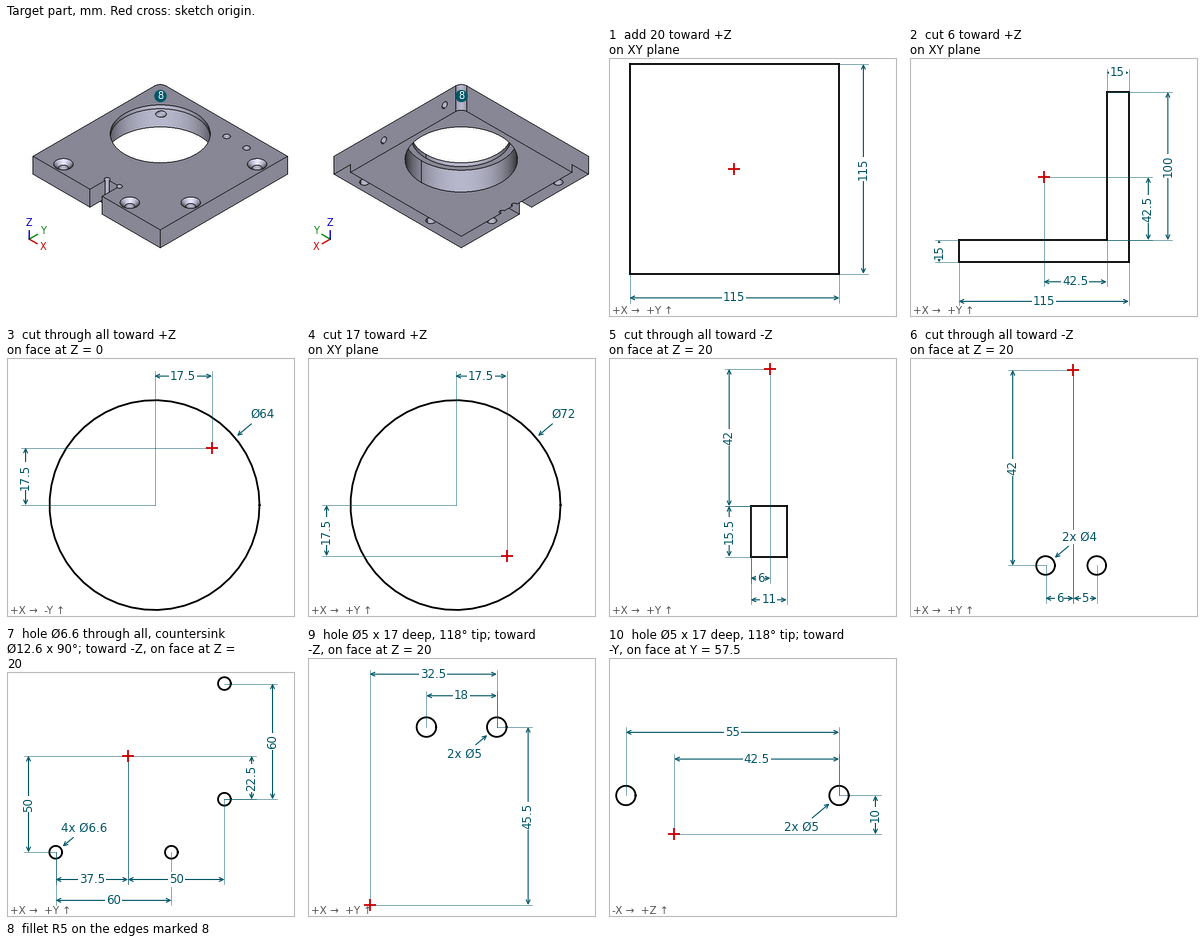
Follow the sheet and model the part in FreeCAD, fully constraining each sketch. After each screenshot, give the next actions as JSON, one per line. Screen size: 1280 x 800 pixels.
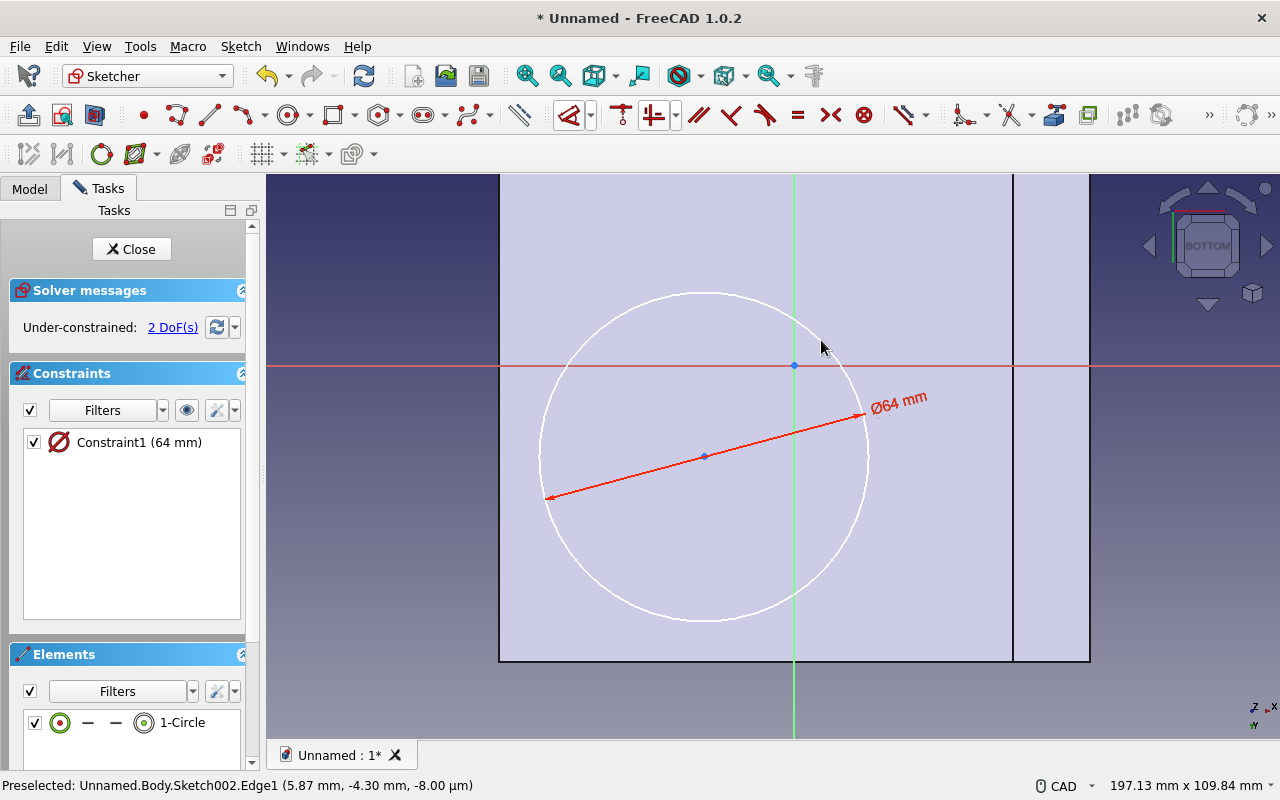
{"action": "left_click", "coordinate": [704, 457]}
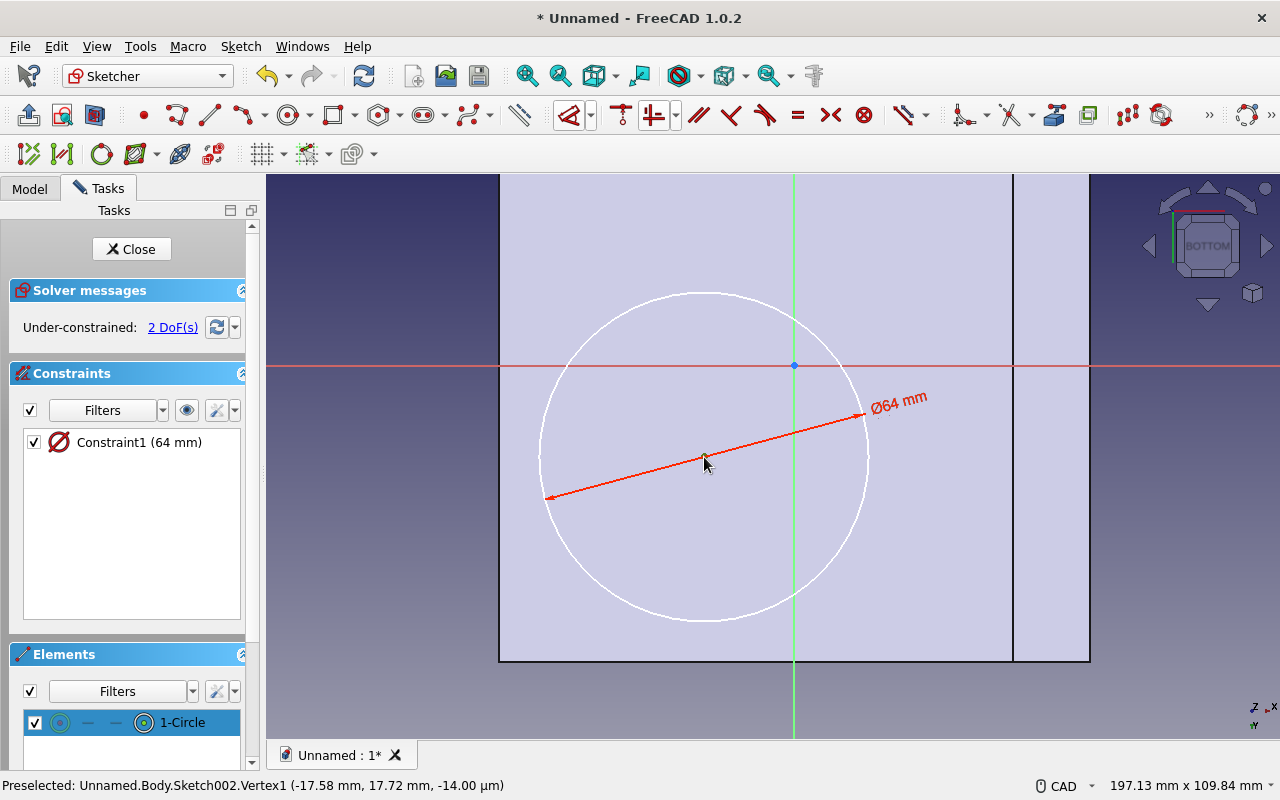
{"action": "key", "text": "l"}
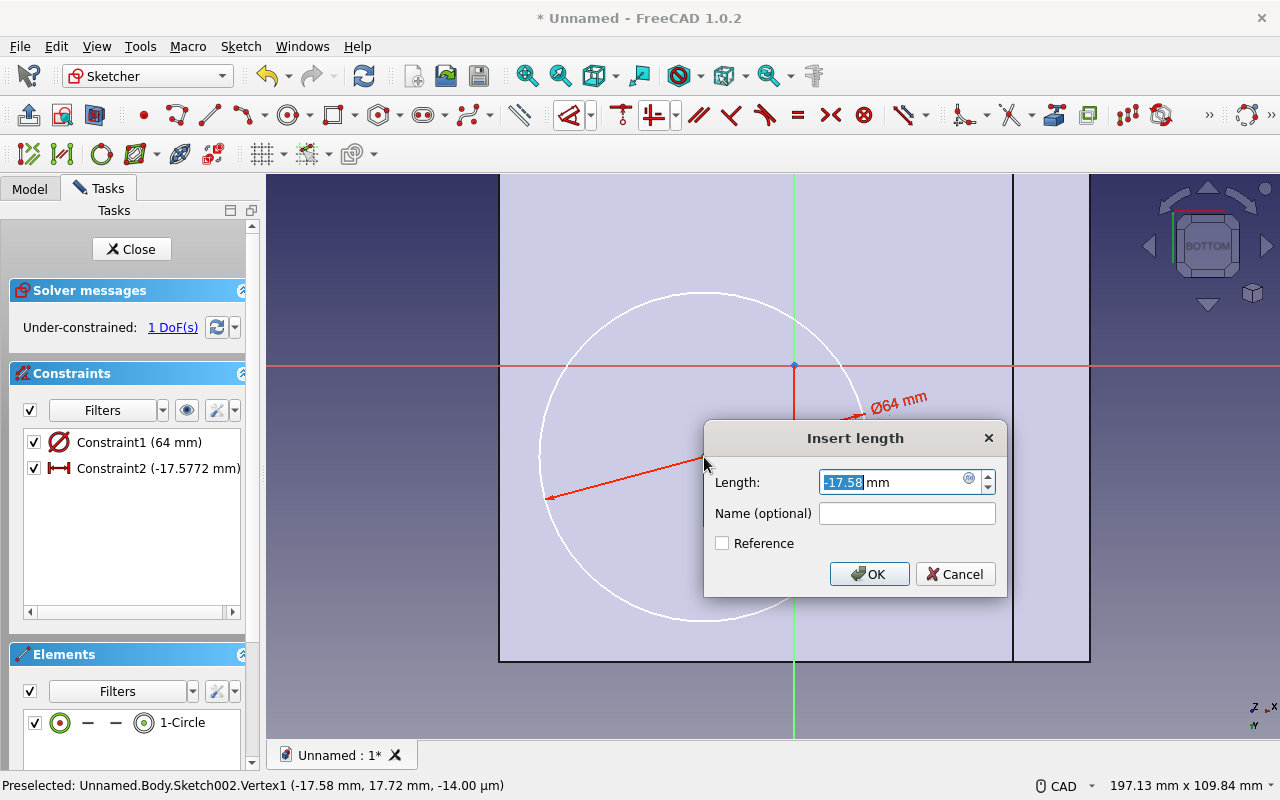
{"action": "type", "text": "-17.5"}
{"action": "key", "text": "Return"}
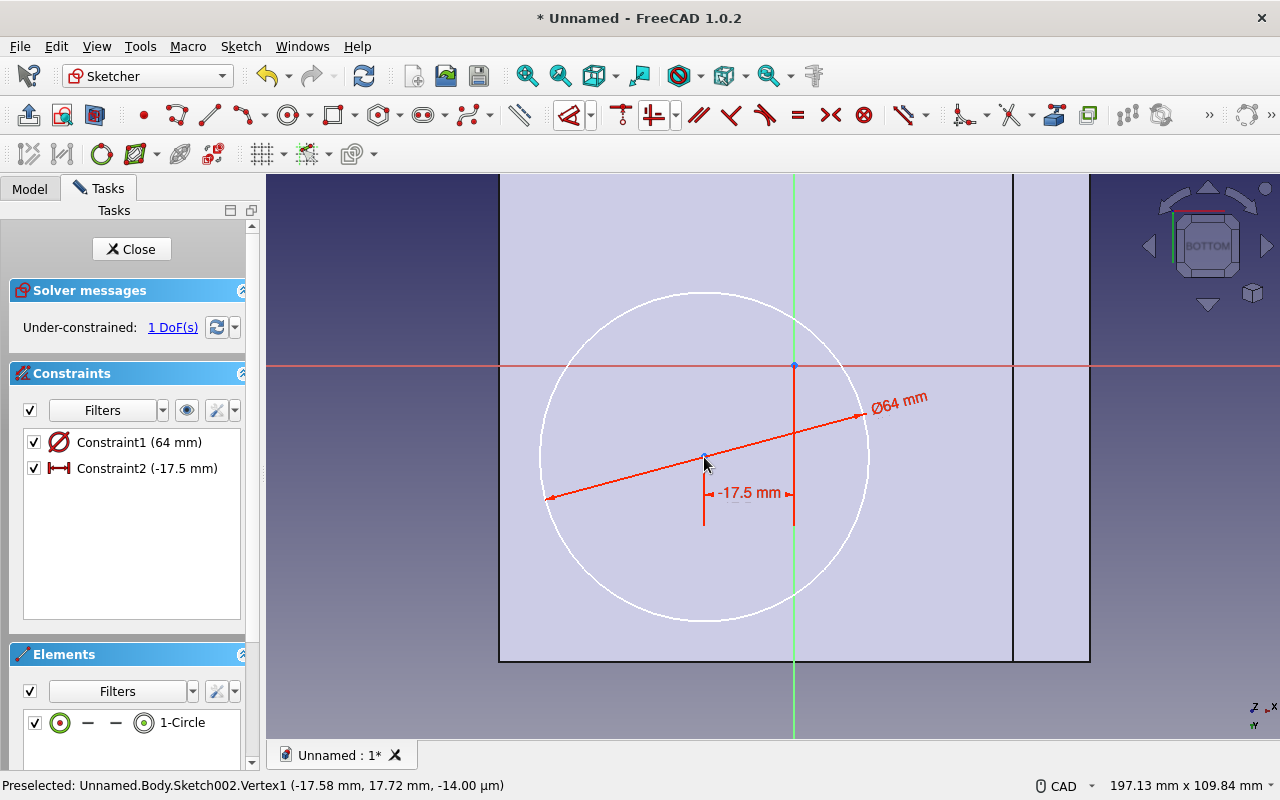
{"action": "left_click", "coordinate": [704, 457]}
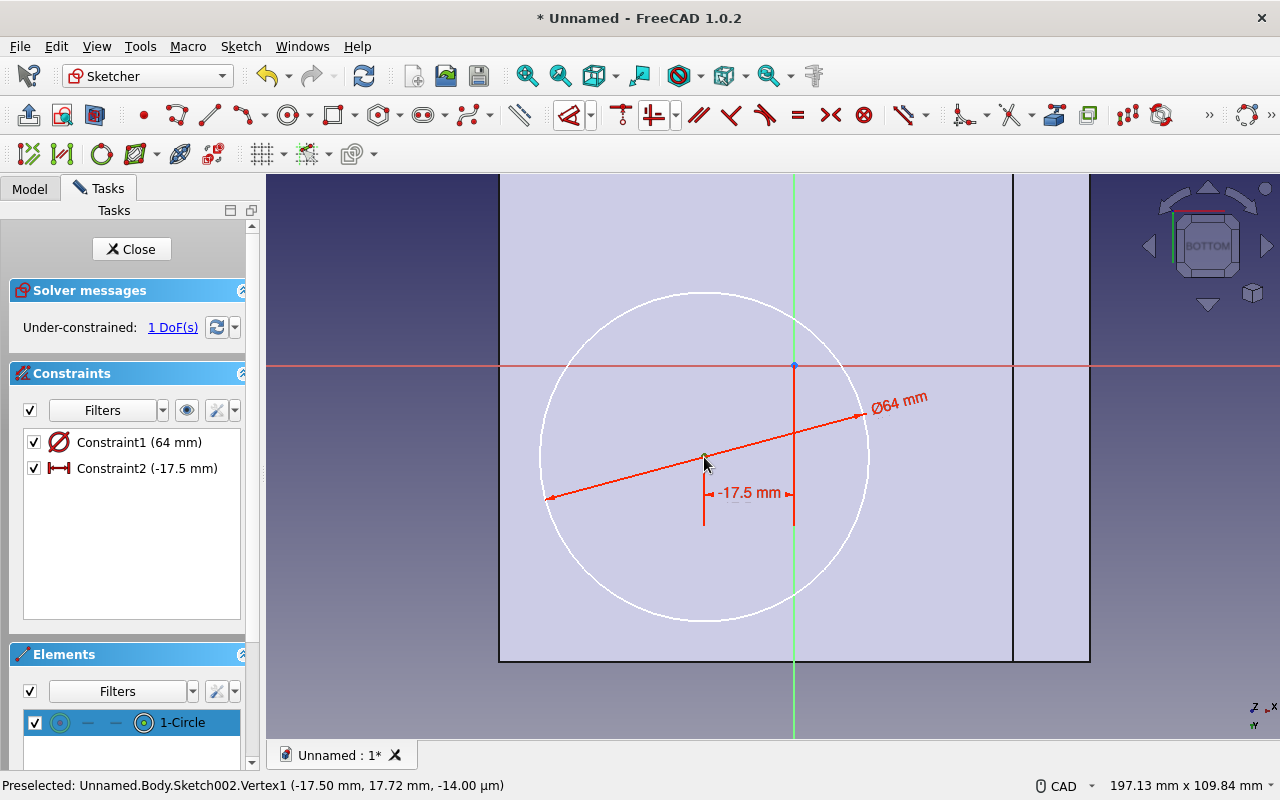
{"action": "key", "text": "i"}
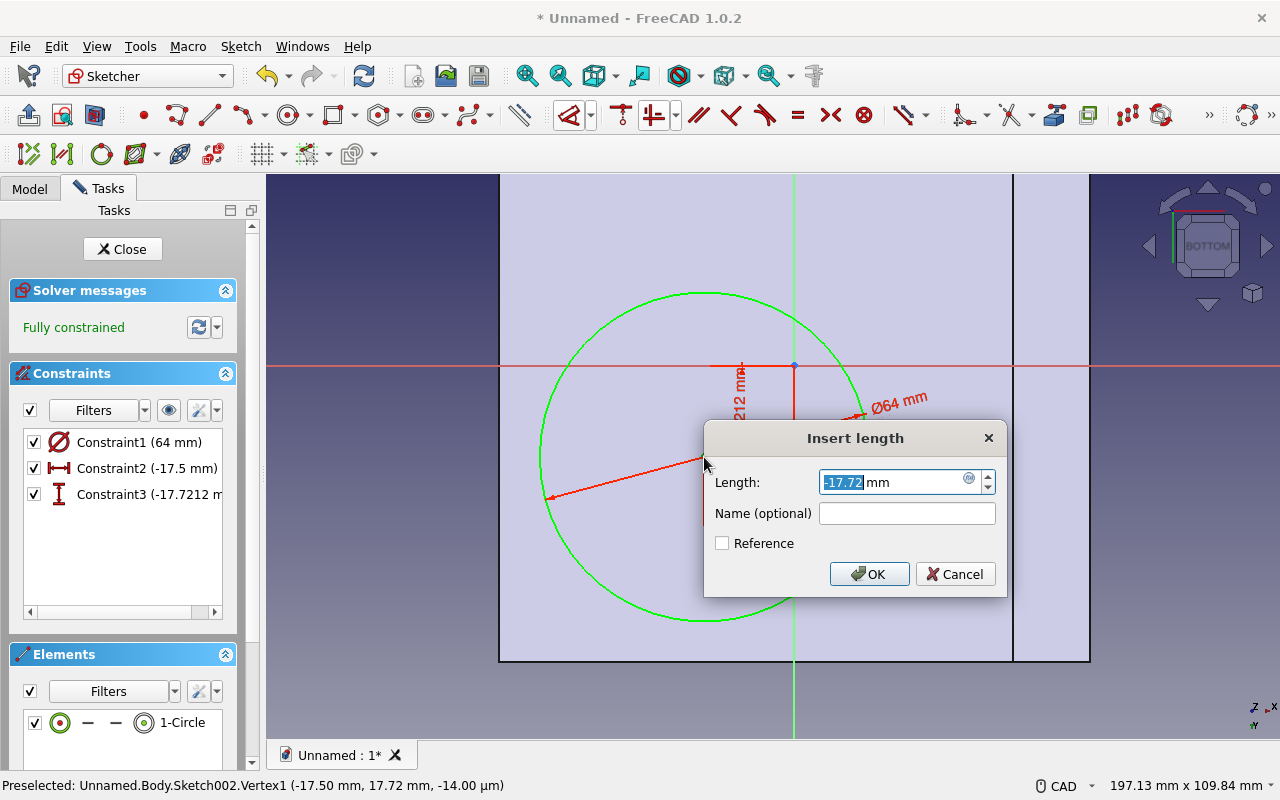
{"action": "type", "text": "-17.5"}
{"action": "key", "text": "Return"}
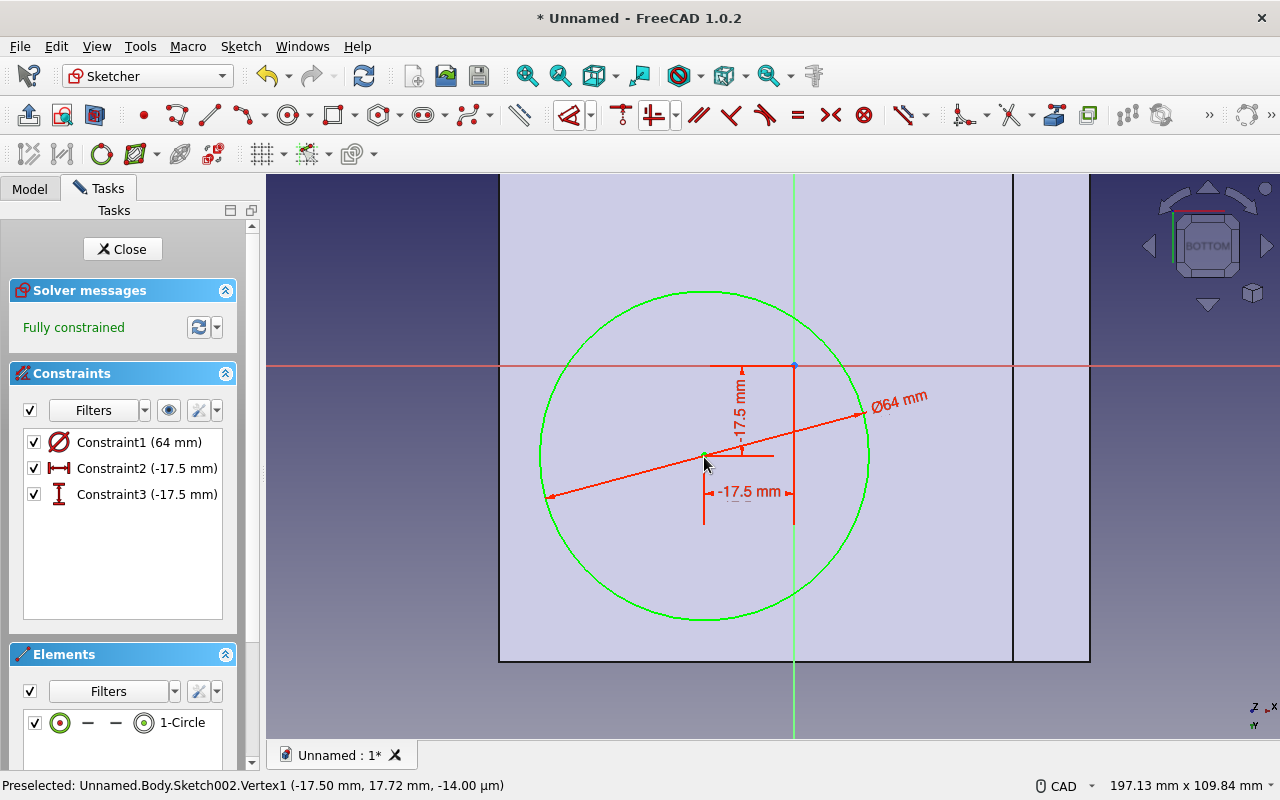
{"action": "left_click", "coordinate": [123, 249]}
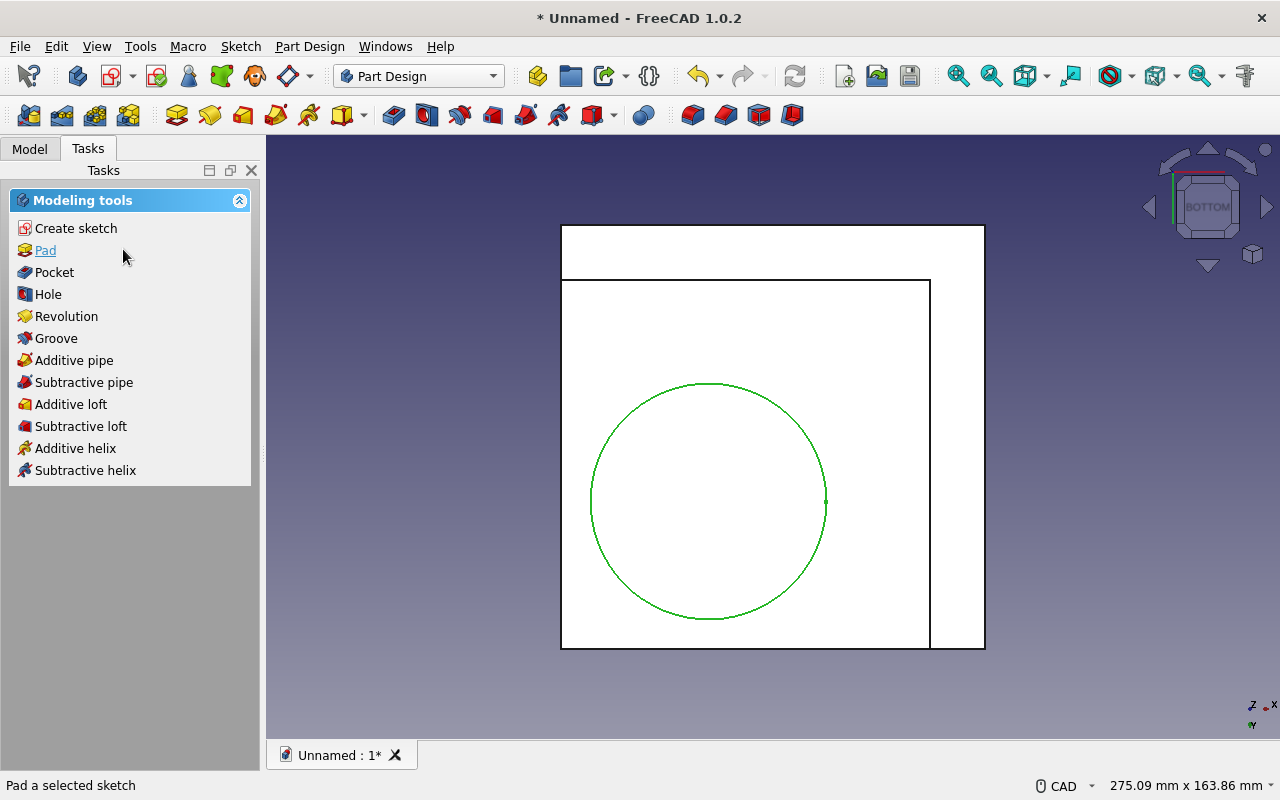
{"action": "left_click", "coordinate": [394, 116]}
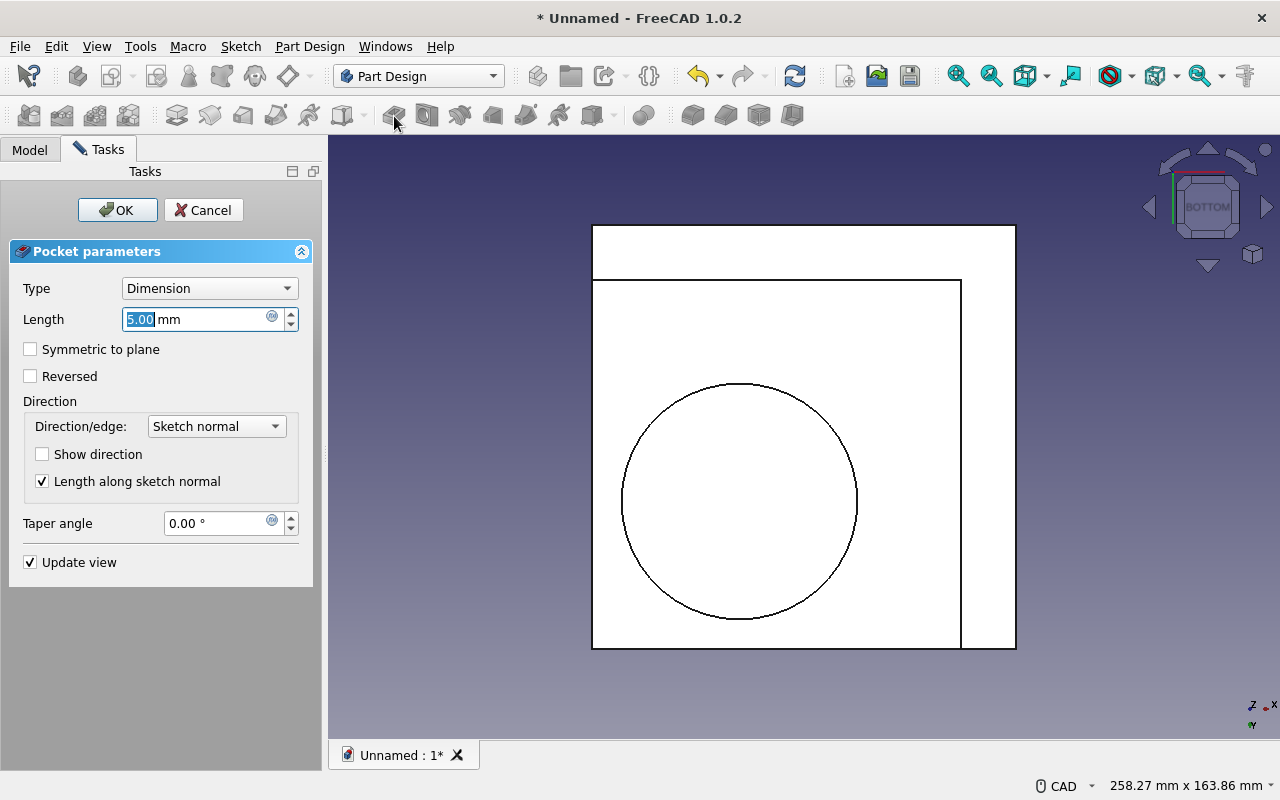
{"action": "left_click", "coordinate": [210, 288]}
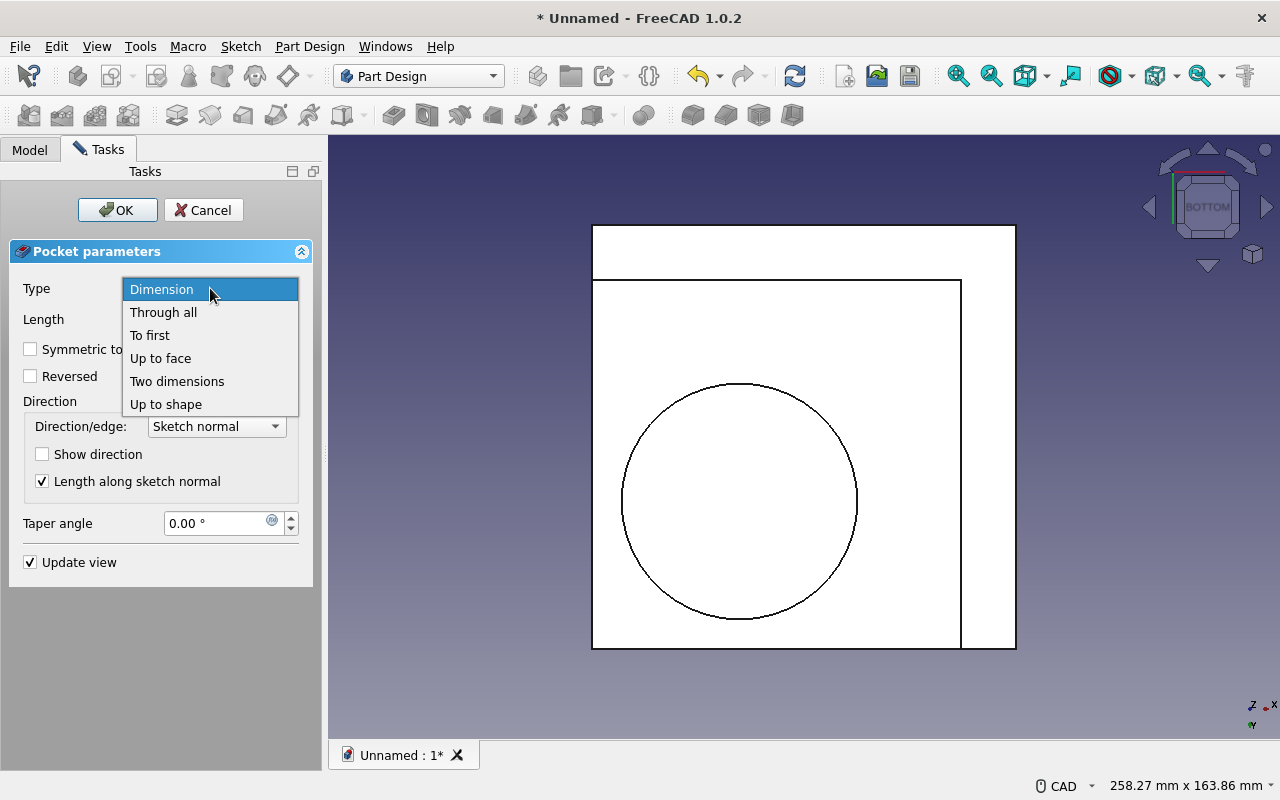
{"action": "left_click", "coordinate": [208, 312]}